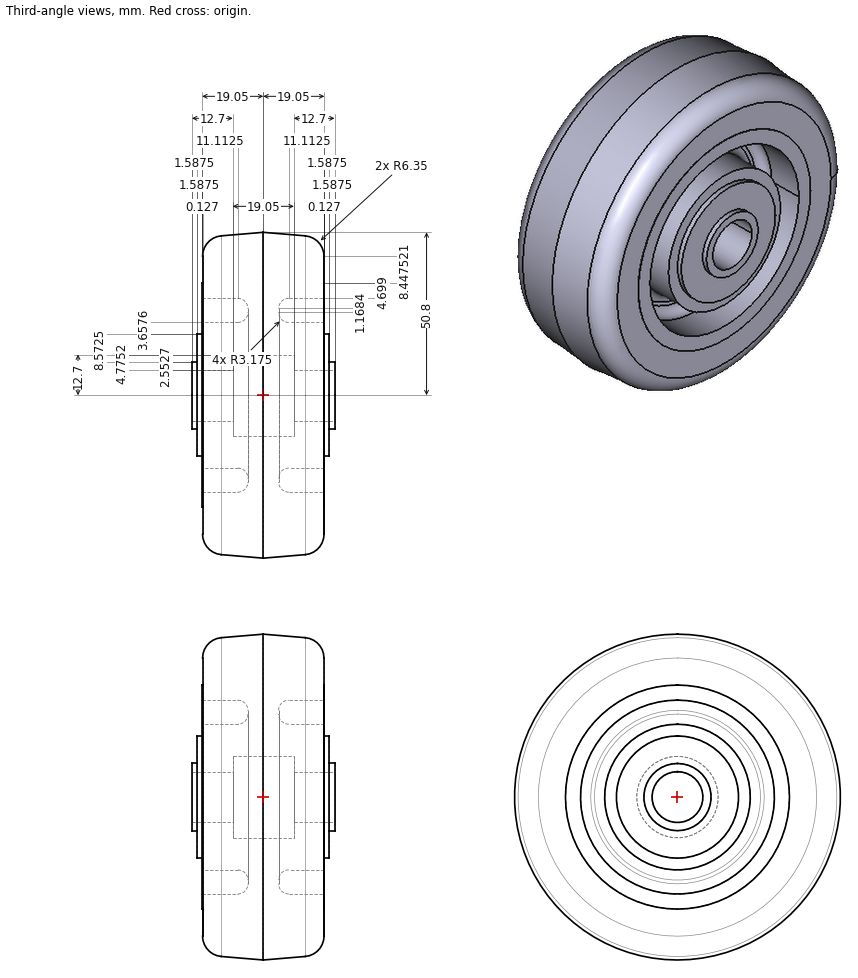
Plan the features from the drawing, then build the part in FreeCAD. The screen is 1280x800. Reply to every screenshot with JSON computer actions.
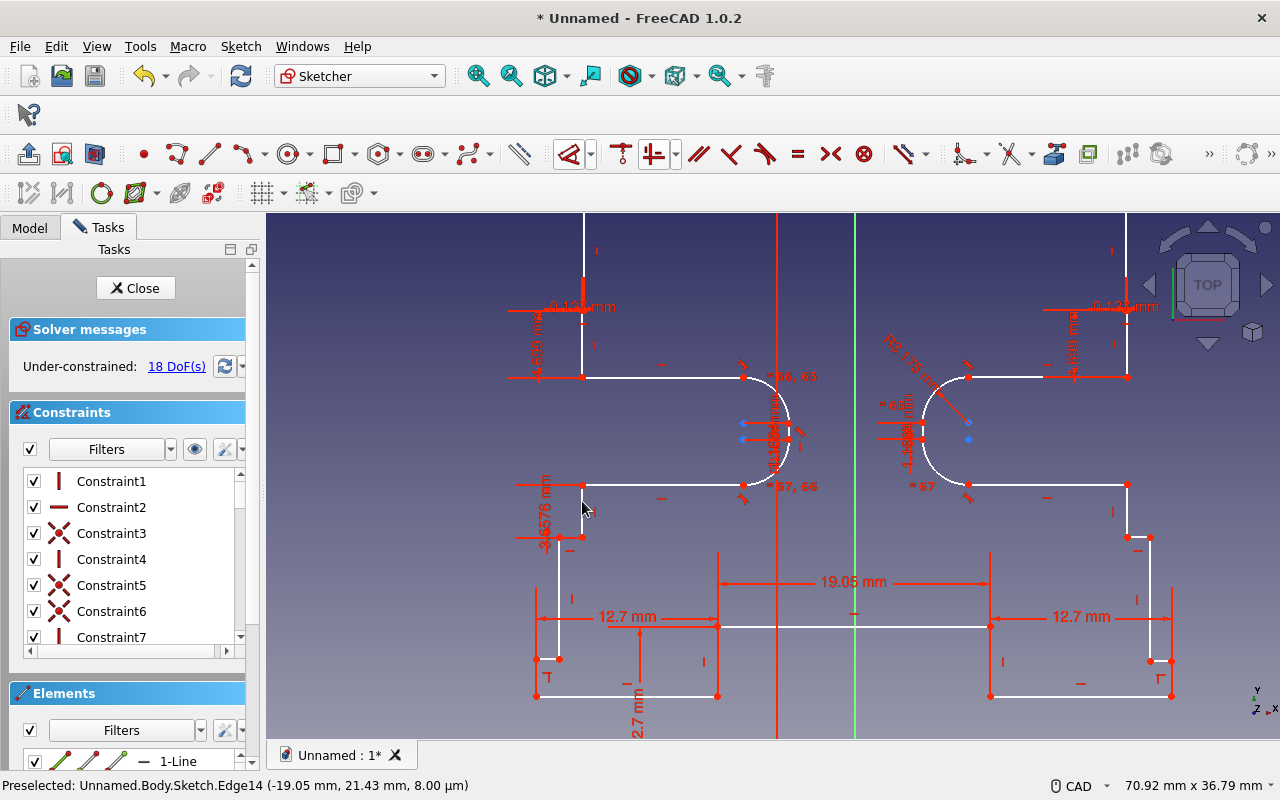
{"action": "scroll", "coordinate": [573, 538], "scroll_direction": "up", "scroll_amount": 3}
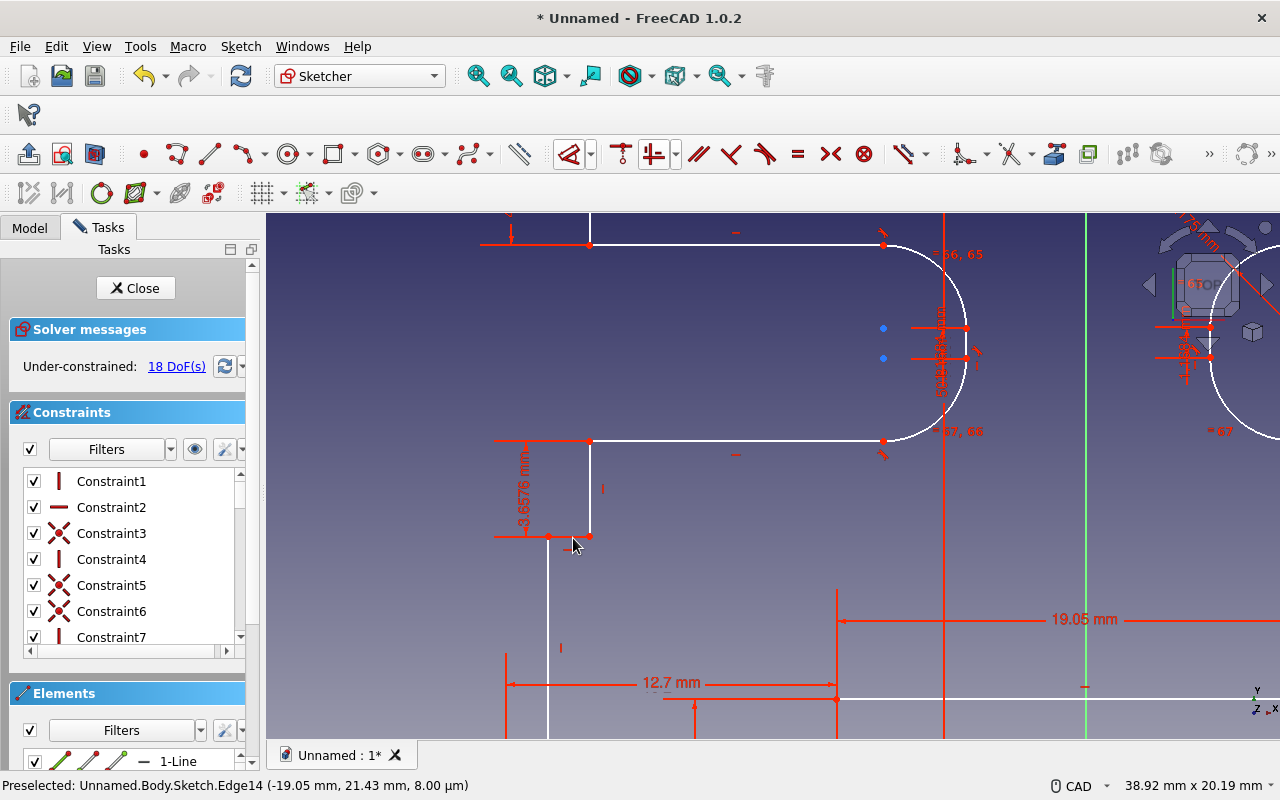
{"action": "left_click", "coordinate": [573, 537]}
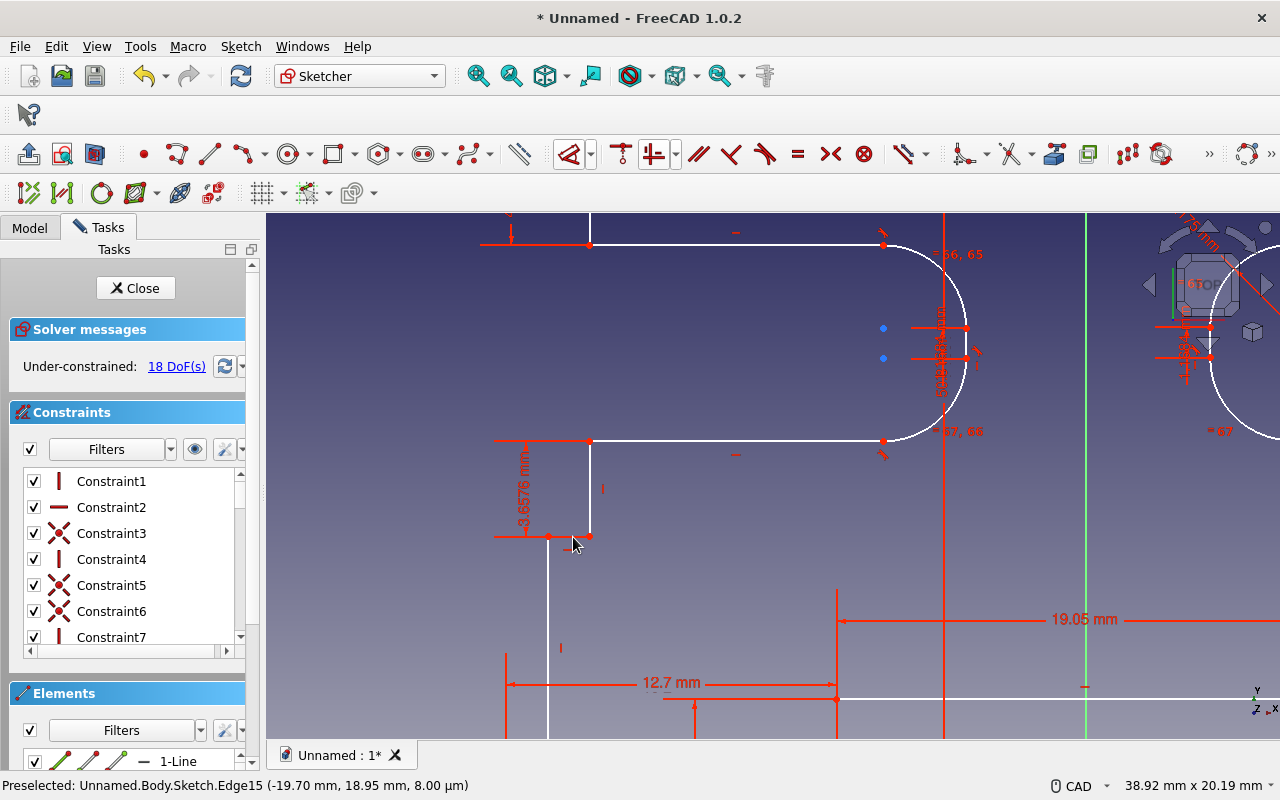
{"action": "left_click", "coordinate": [590, 154]}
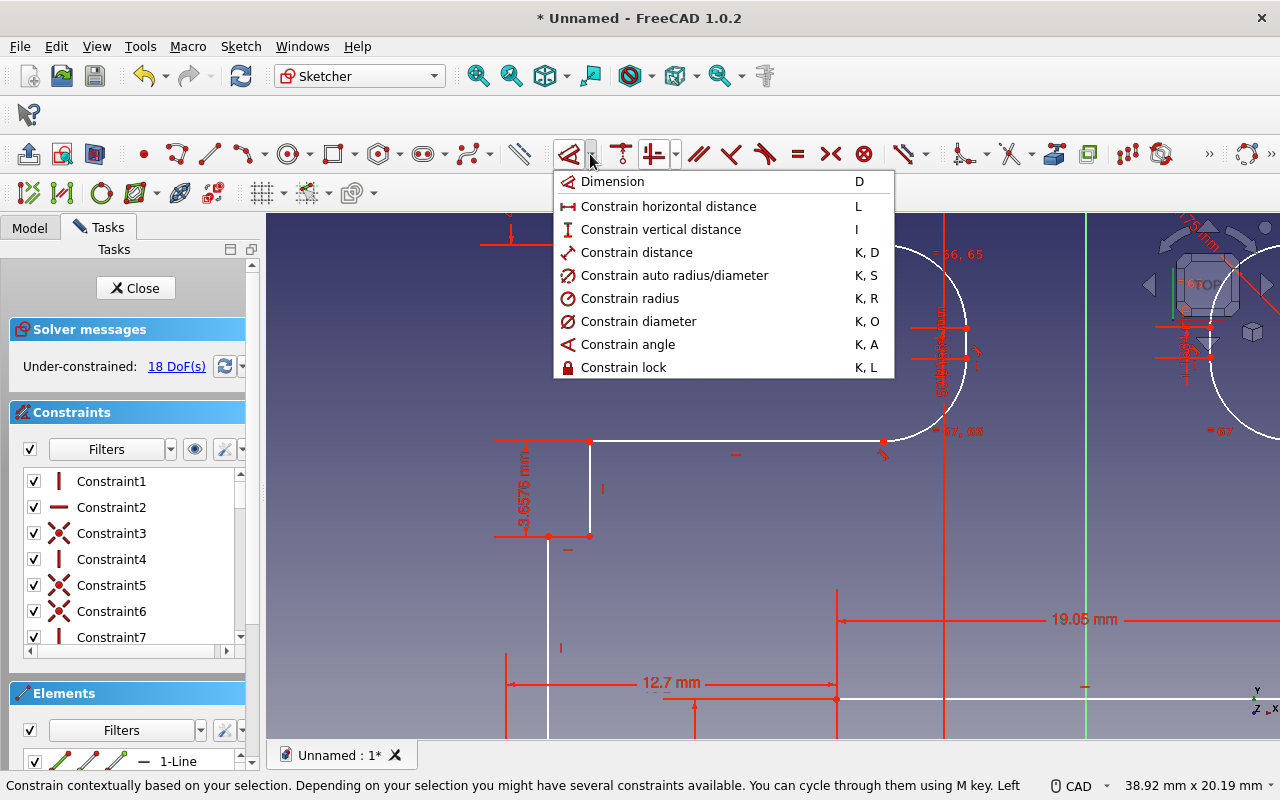
{"action": "left_click", "coordinate": [724, 206]}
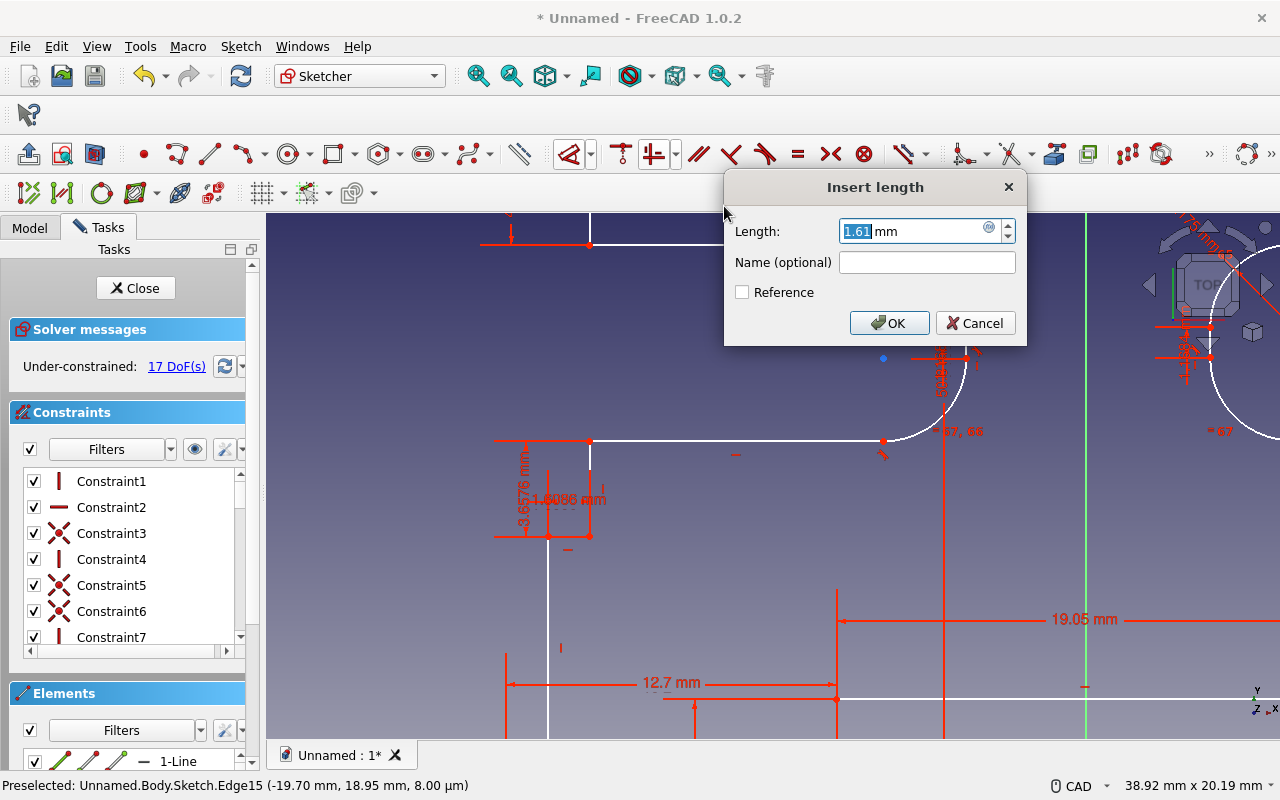
{"action": "type", "text": "1.5875"}
{"action": "key", "text": "Return"}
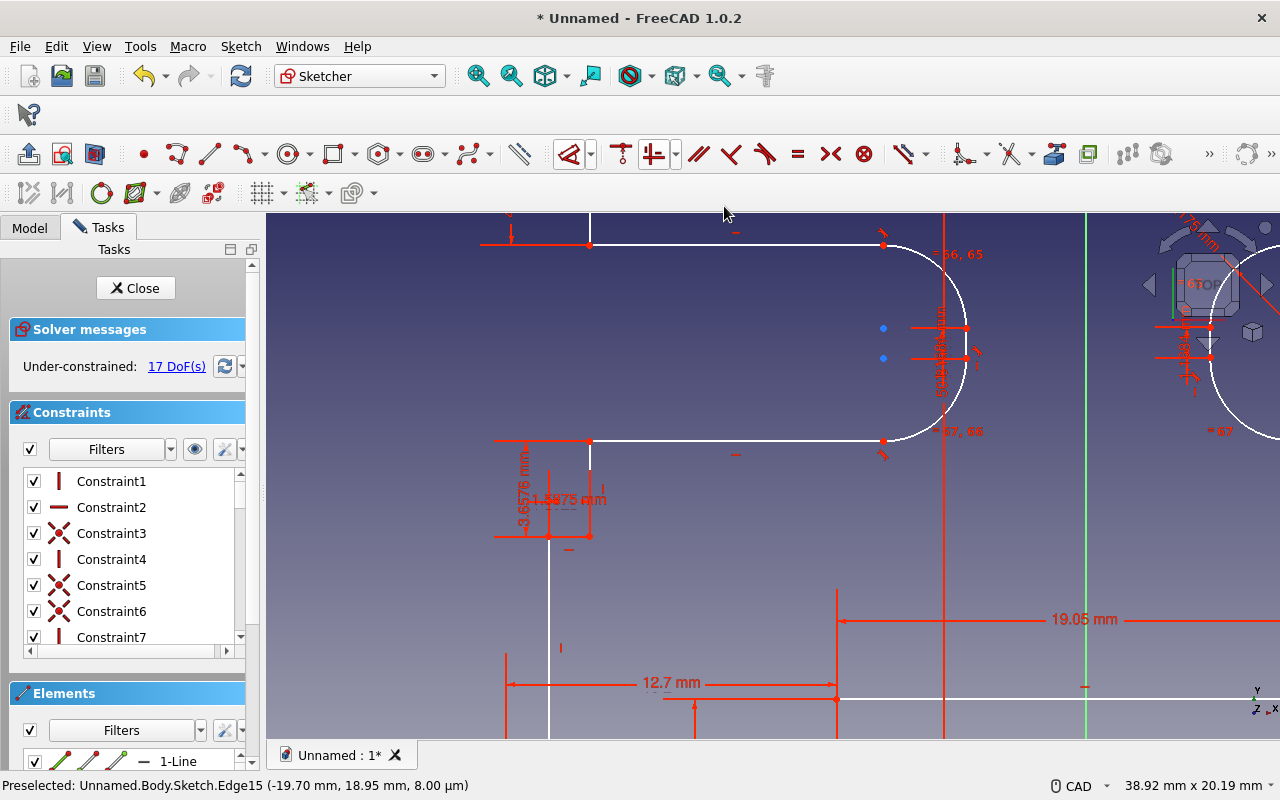
{"action": "scroll", "coordinate": [580, 511], "scroll_direction": "down", "scroll_amount": 7}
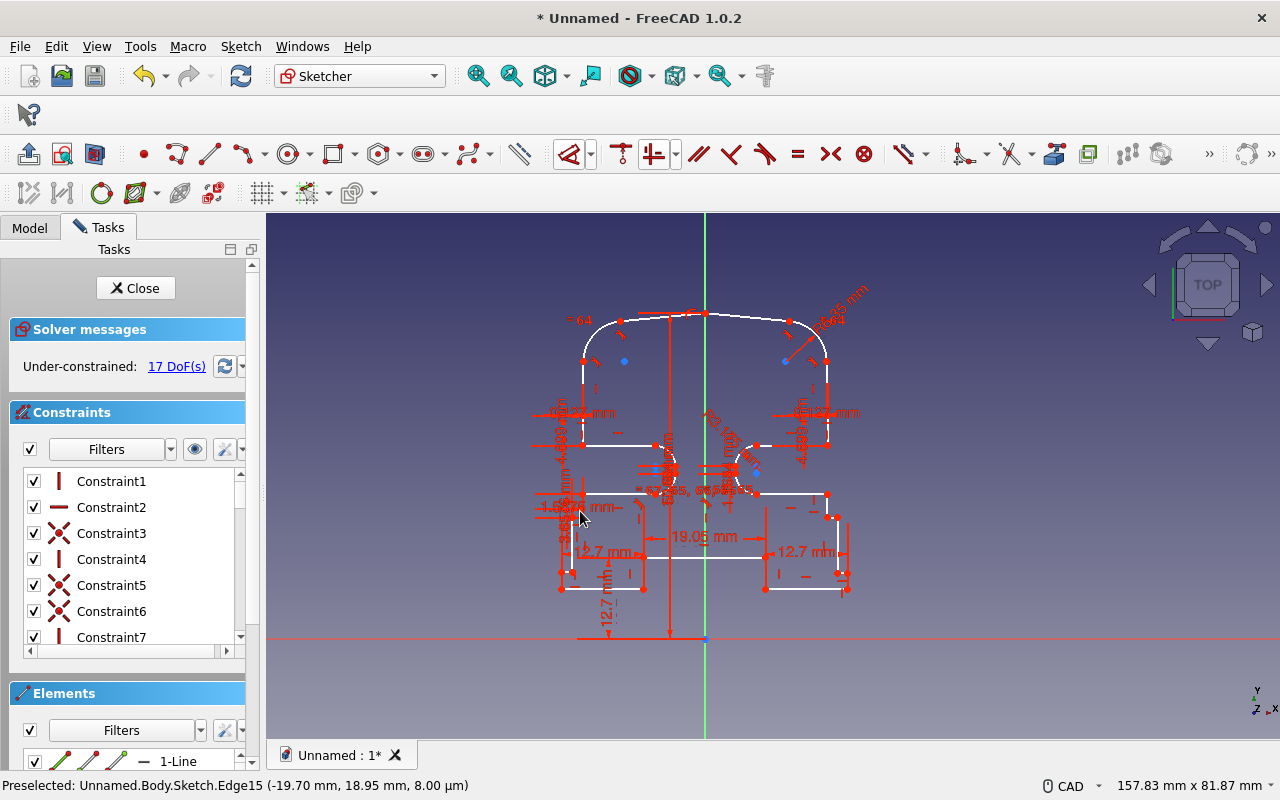
{"action": "left_click", "coordinate": [572, 556]}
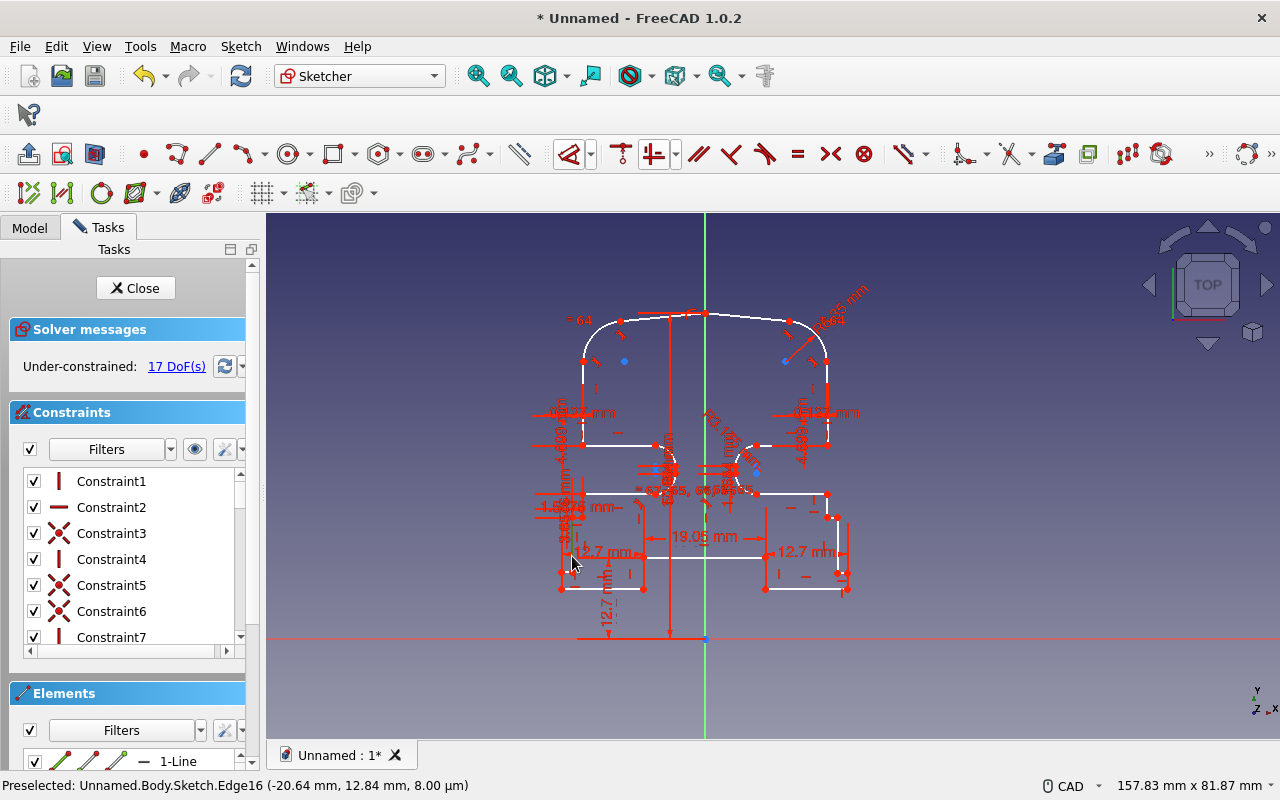
{"action": "key", "text": "i"}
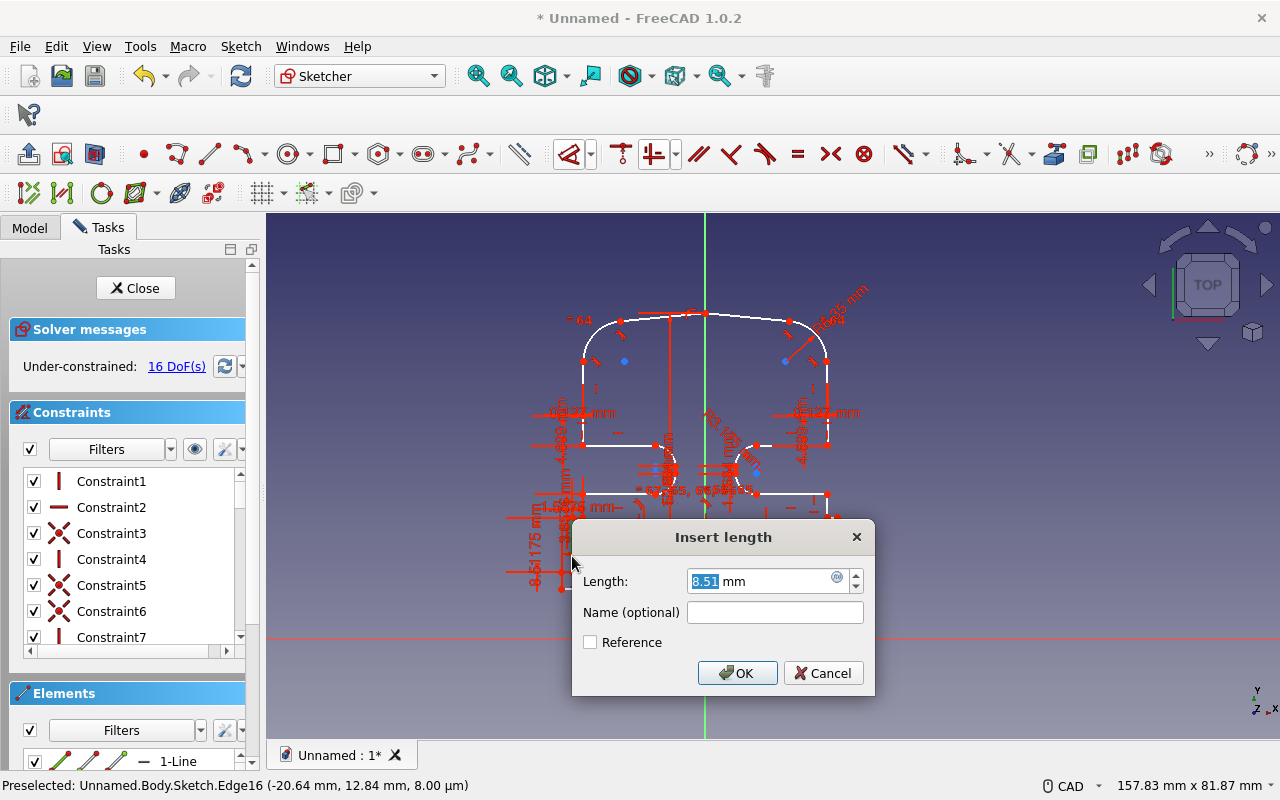
{"action": "type", "text": "8.5725"}
{"action": "key", "text": "Return"}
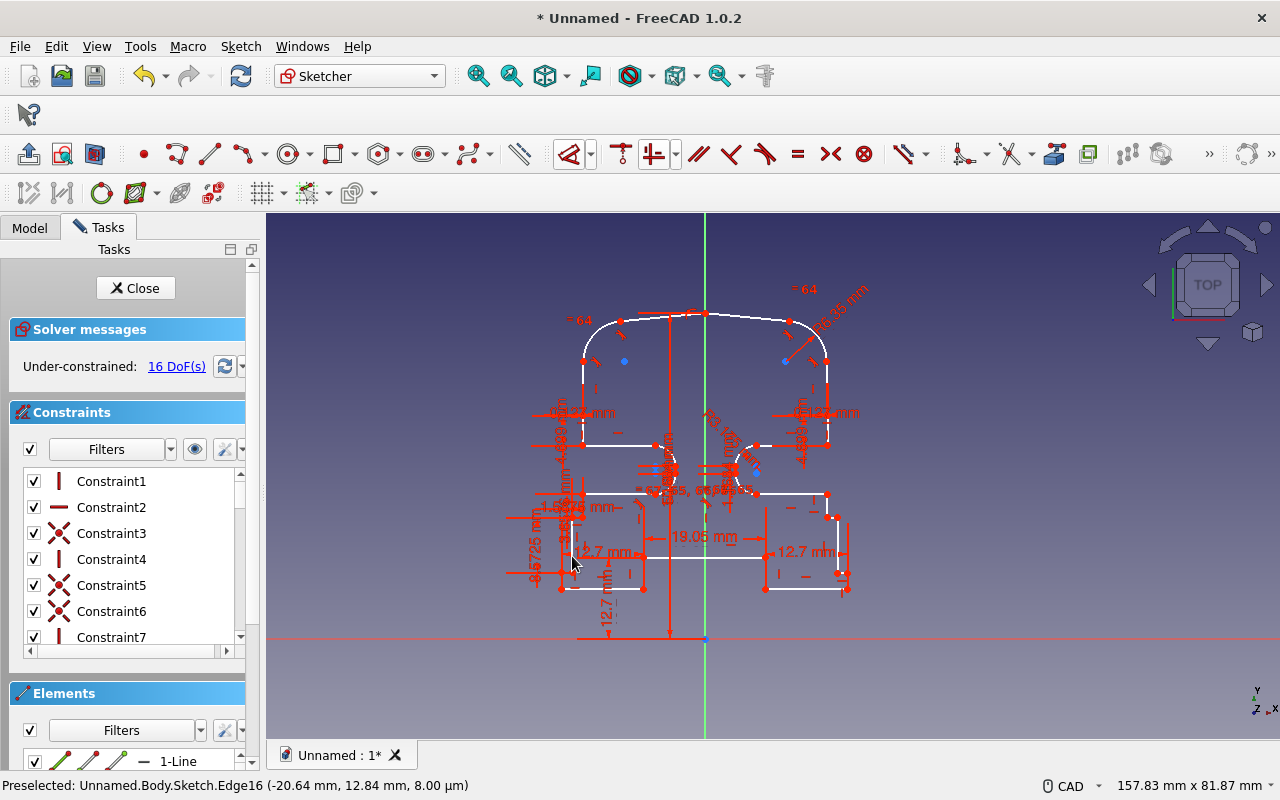
{"action": "scroll", "coordinate": [567, 573], "scroll_direction": "up", "scroll_amount": 7}